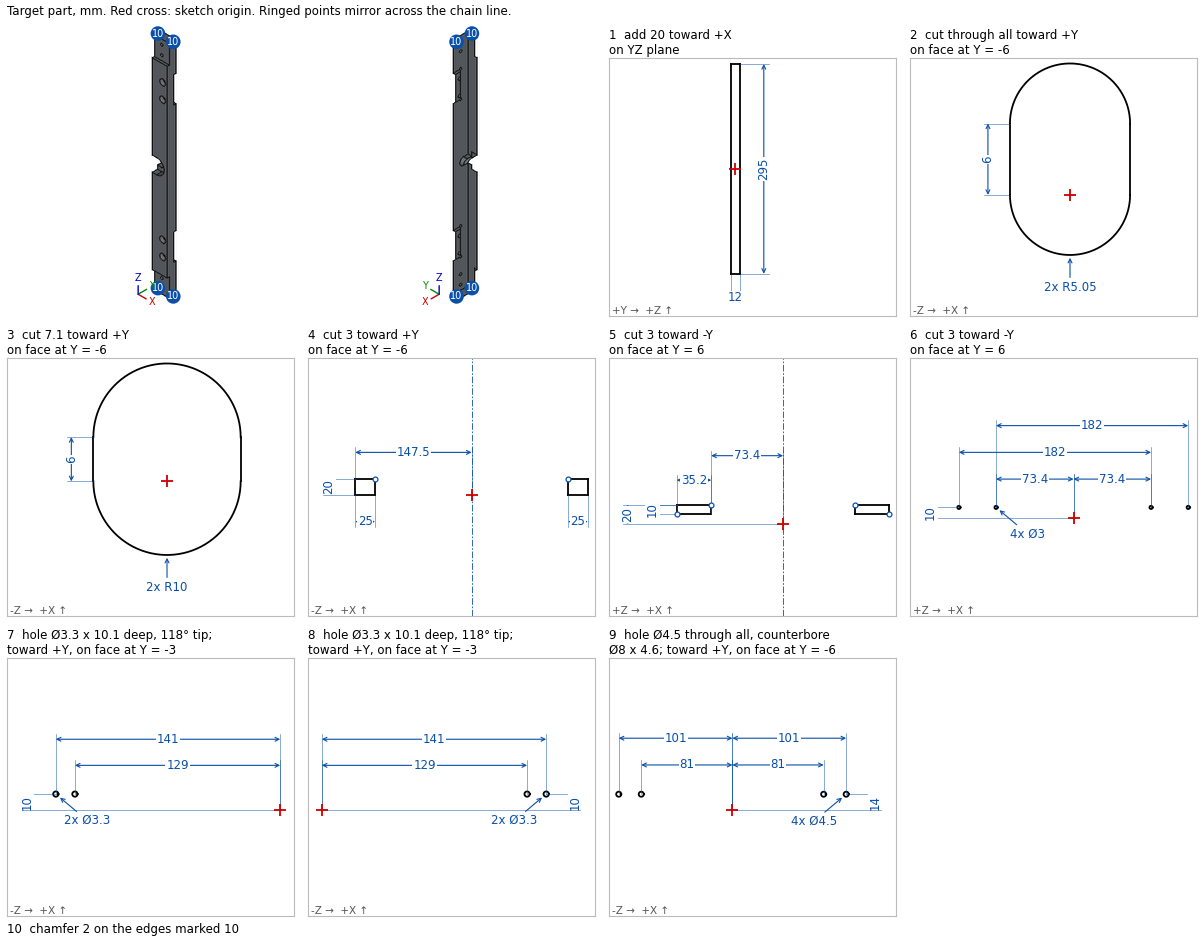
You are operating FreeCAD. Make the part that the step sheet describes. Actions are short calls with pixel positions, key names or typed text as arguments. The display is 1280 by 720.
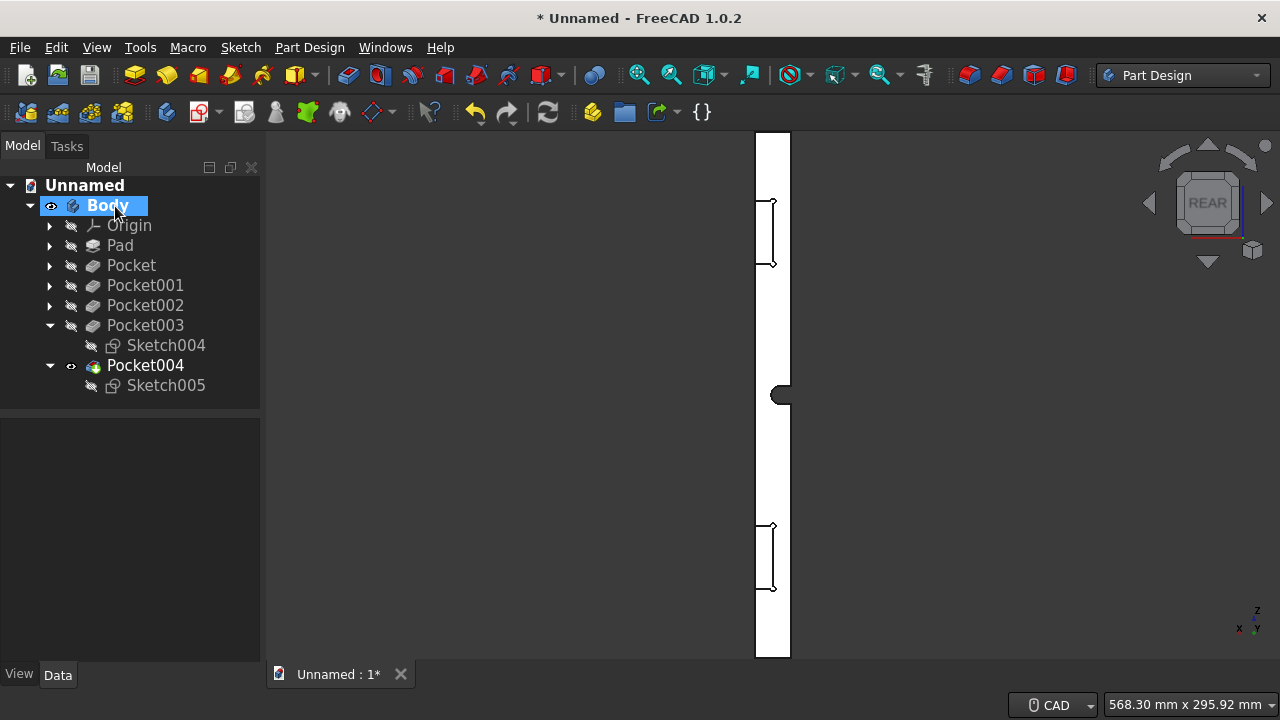
key(0)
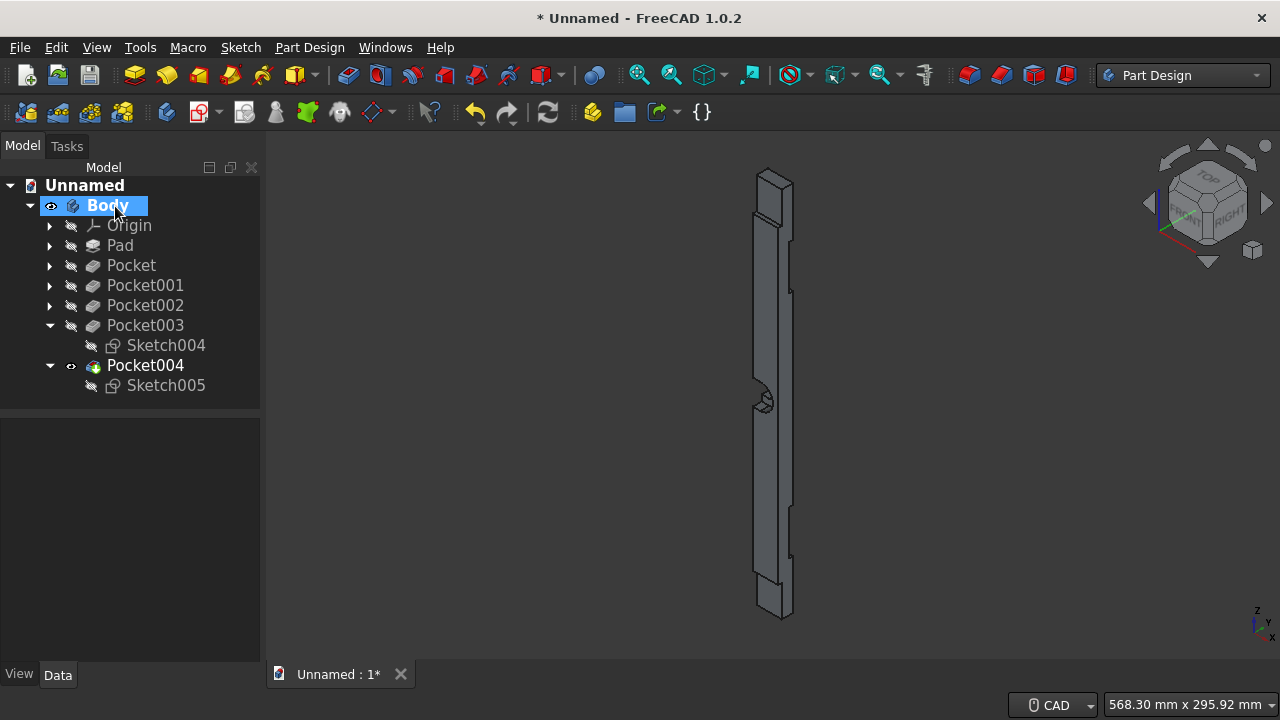
click(769, 593)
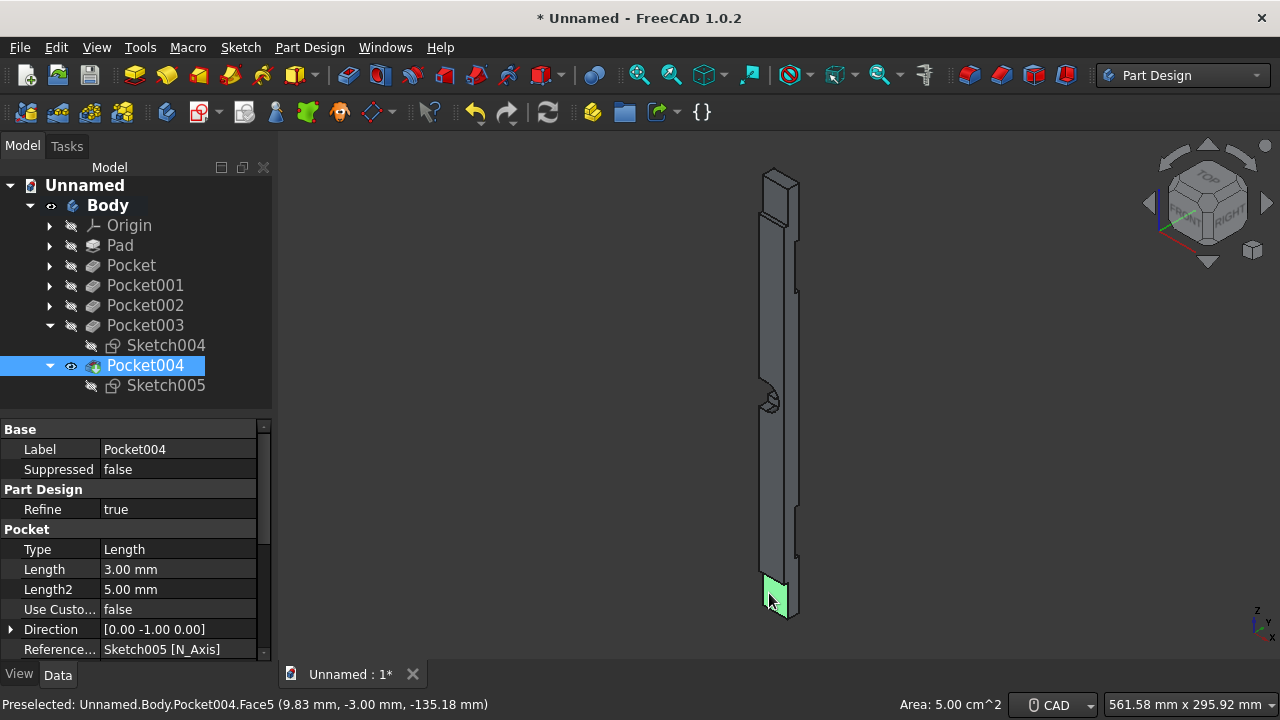
click(200, 112)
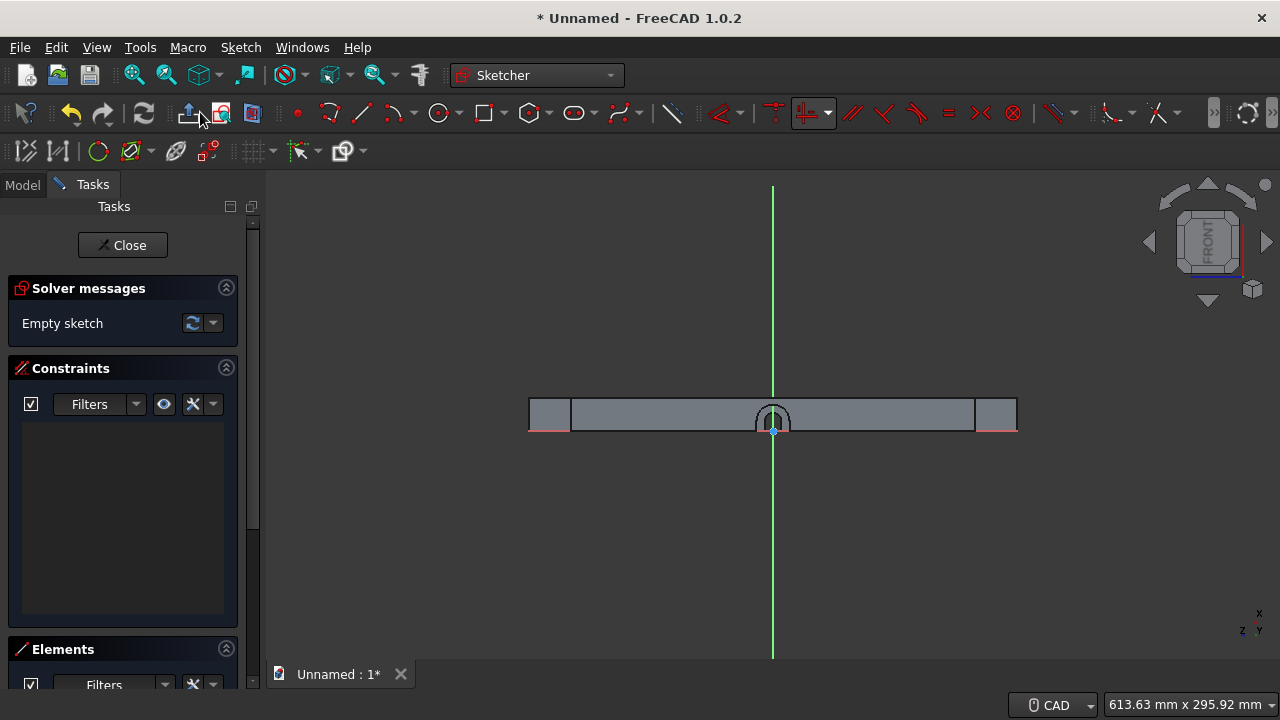
click(254, 114)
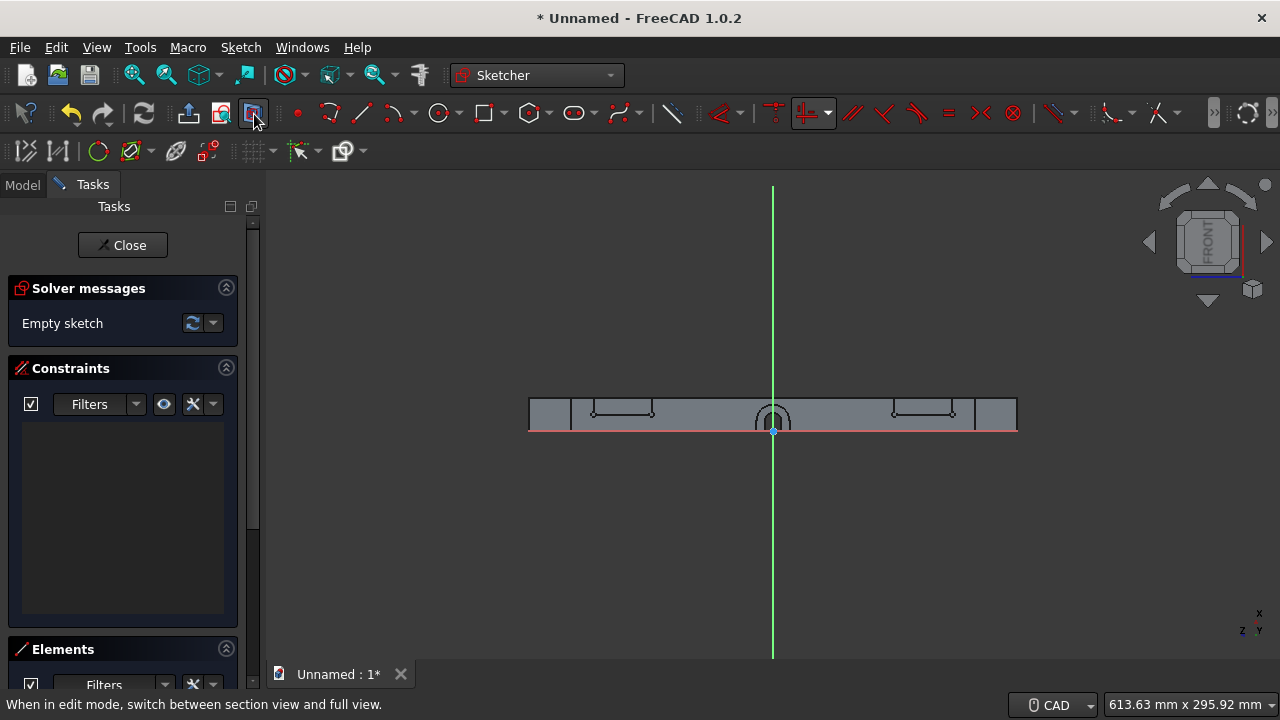
scroll(542, 415, up, 15)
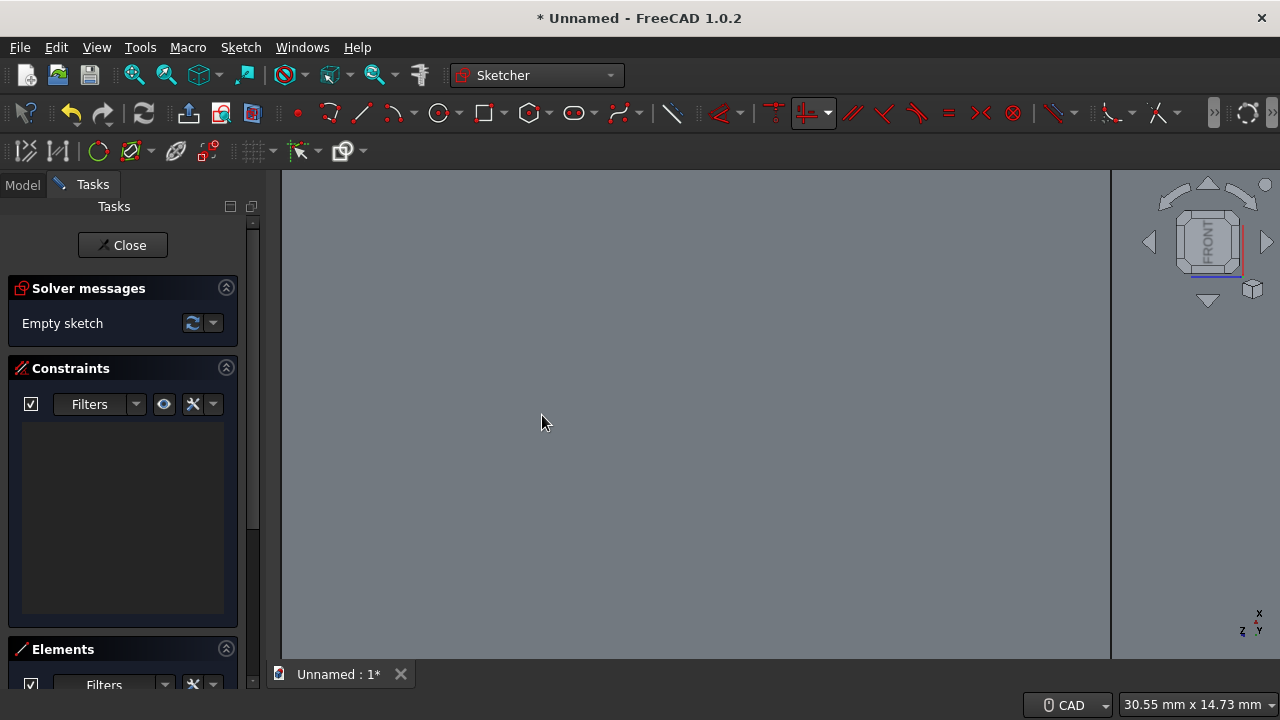
click(440, 114)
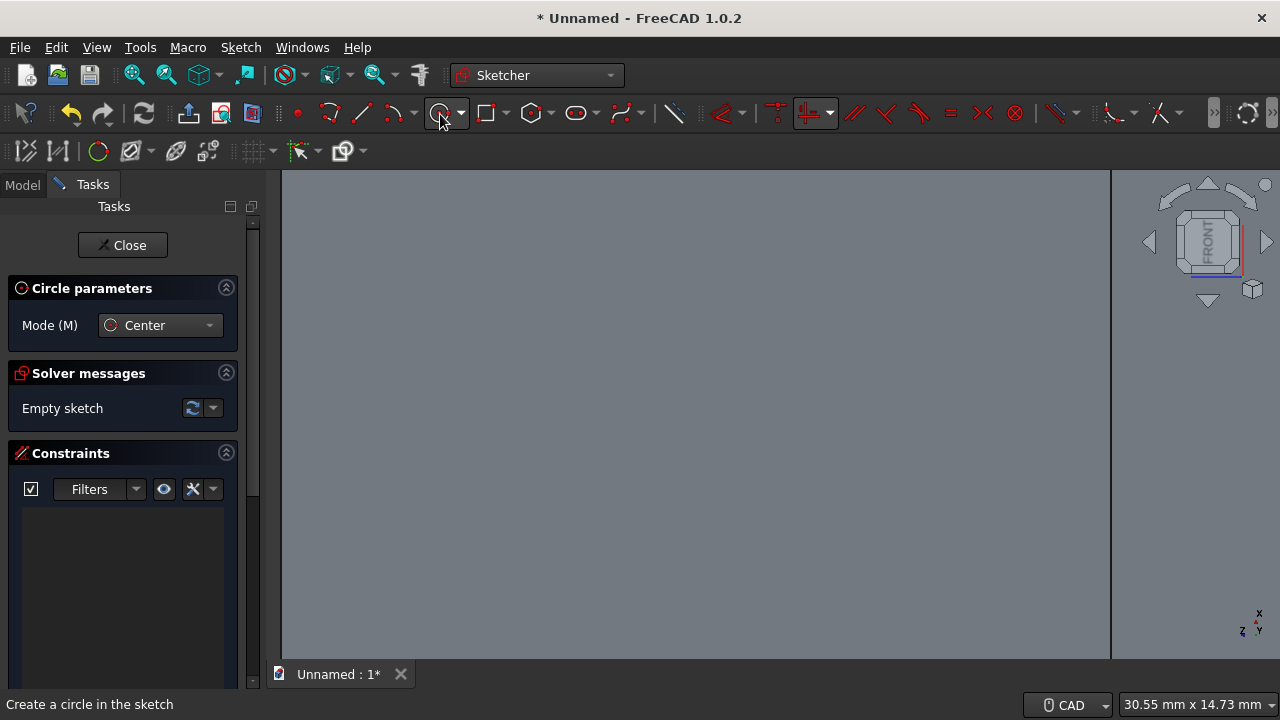
click(497, 395)
click(535, 357)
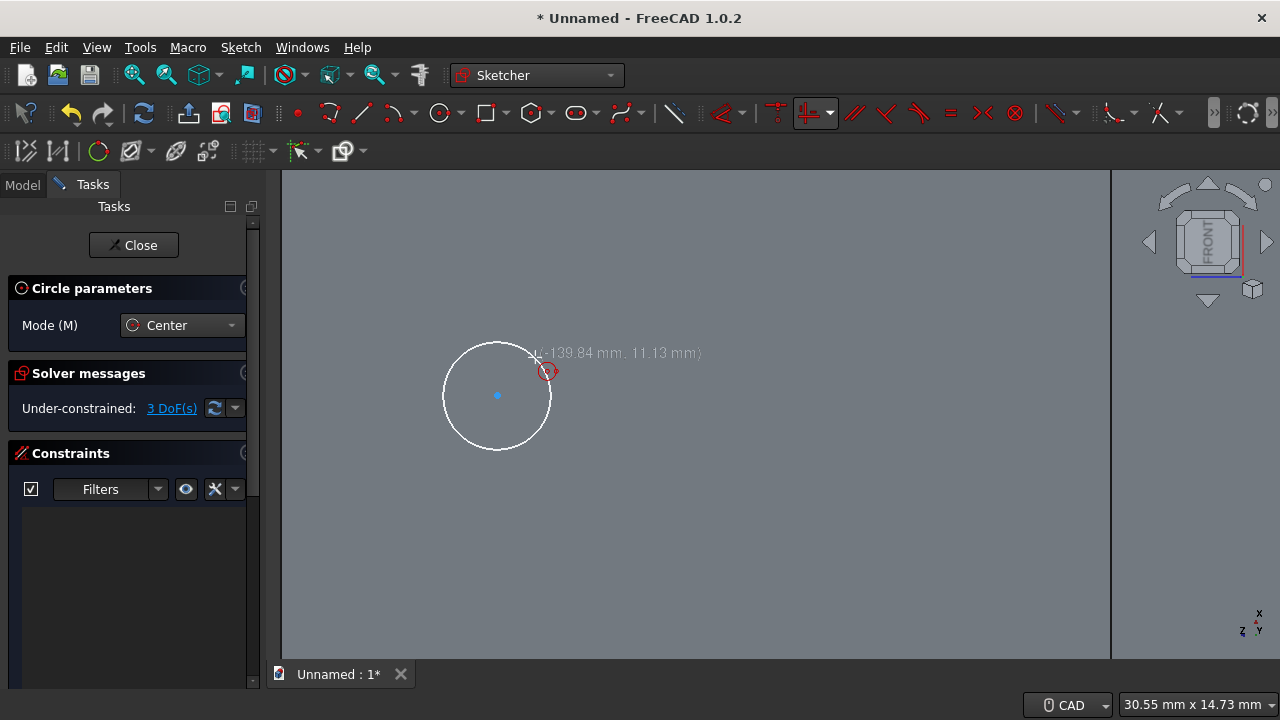
click(895, 395)
click(934, 357)
key(Escape)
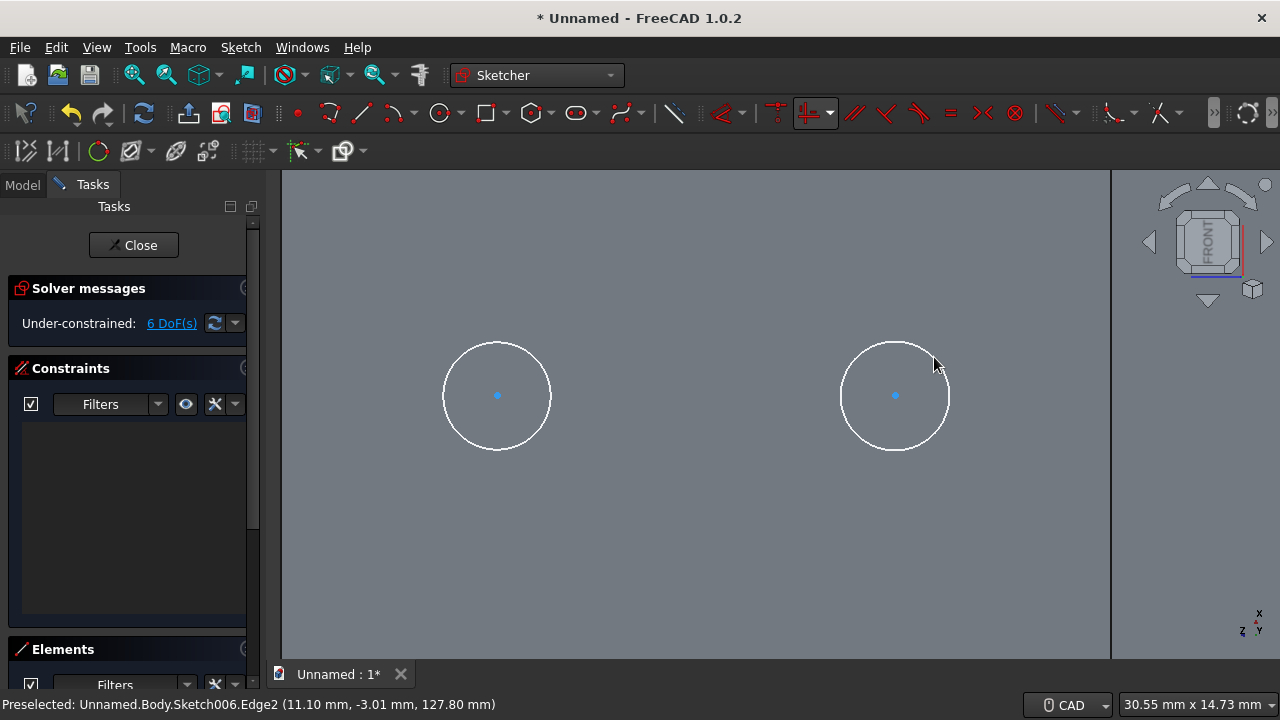
click(535, 358)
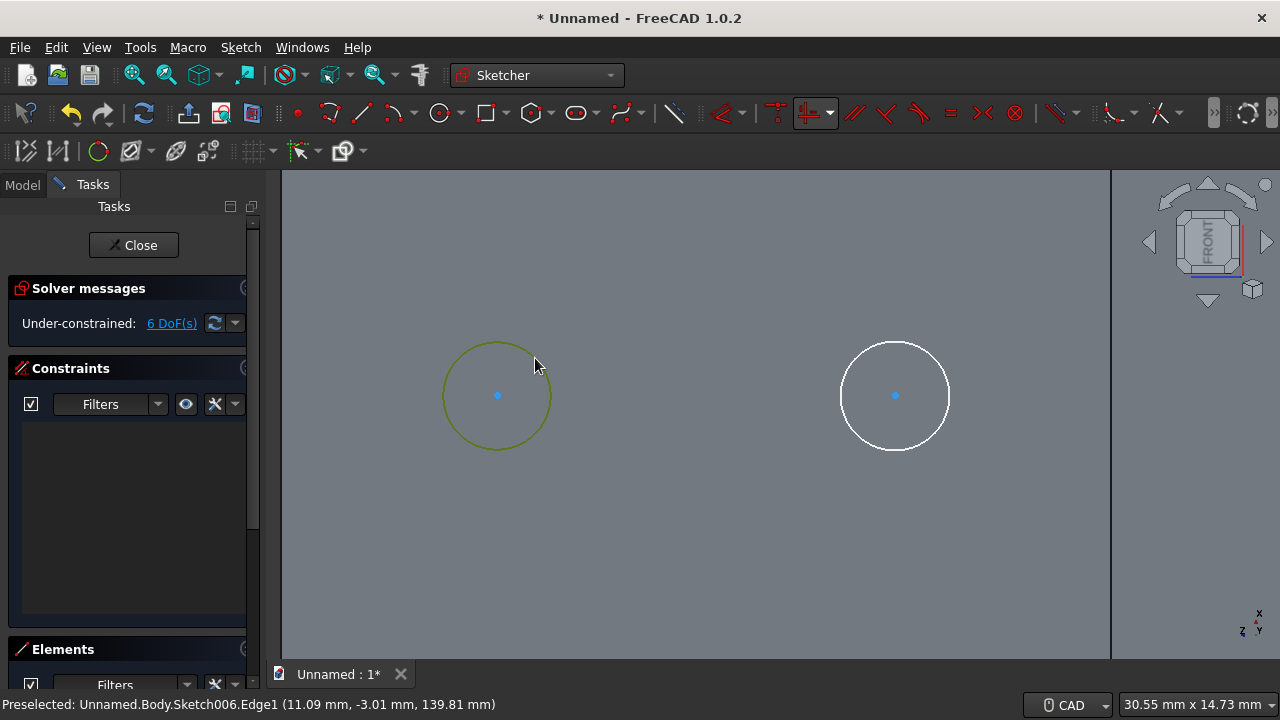
click(933, 357)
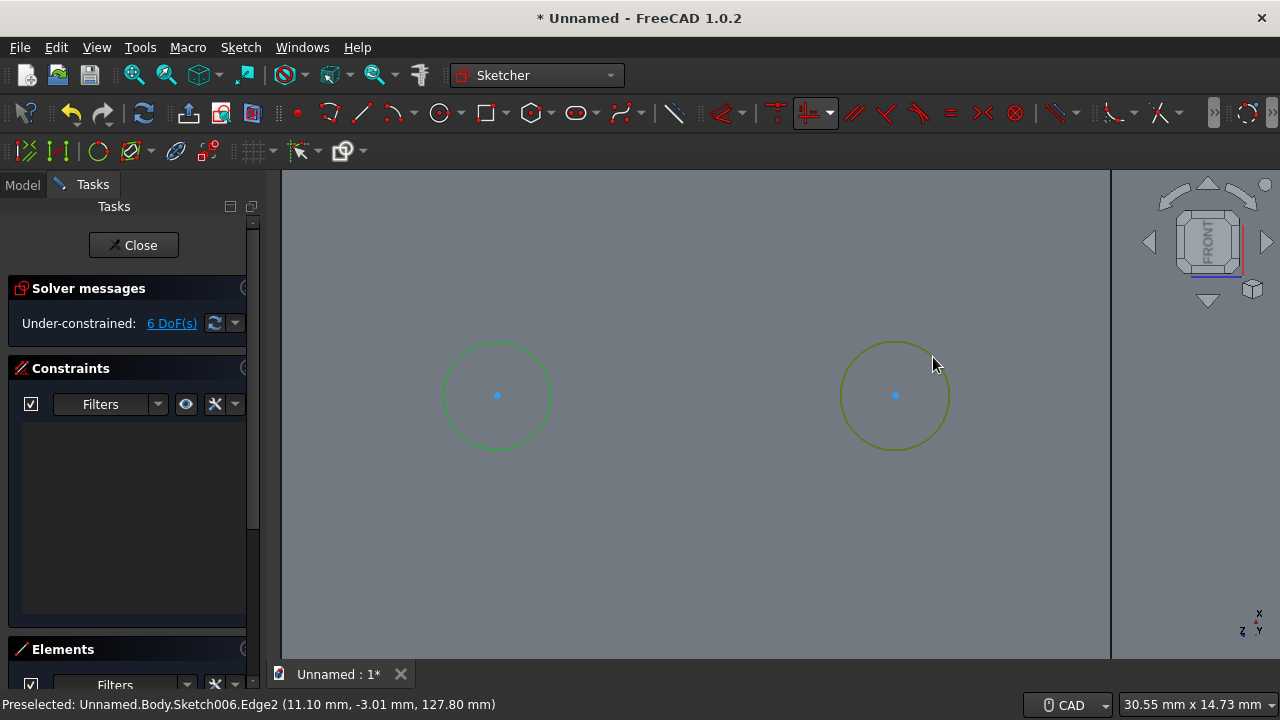
click(952, 114)